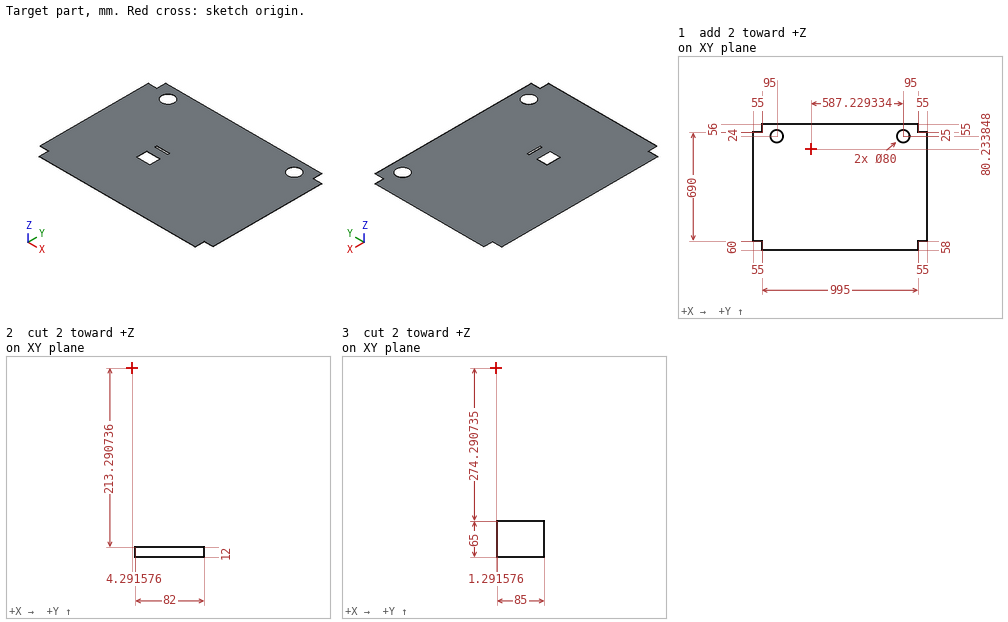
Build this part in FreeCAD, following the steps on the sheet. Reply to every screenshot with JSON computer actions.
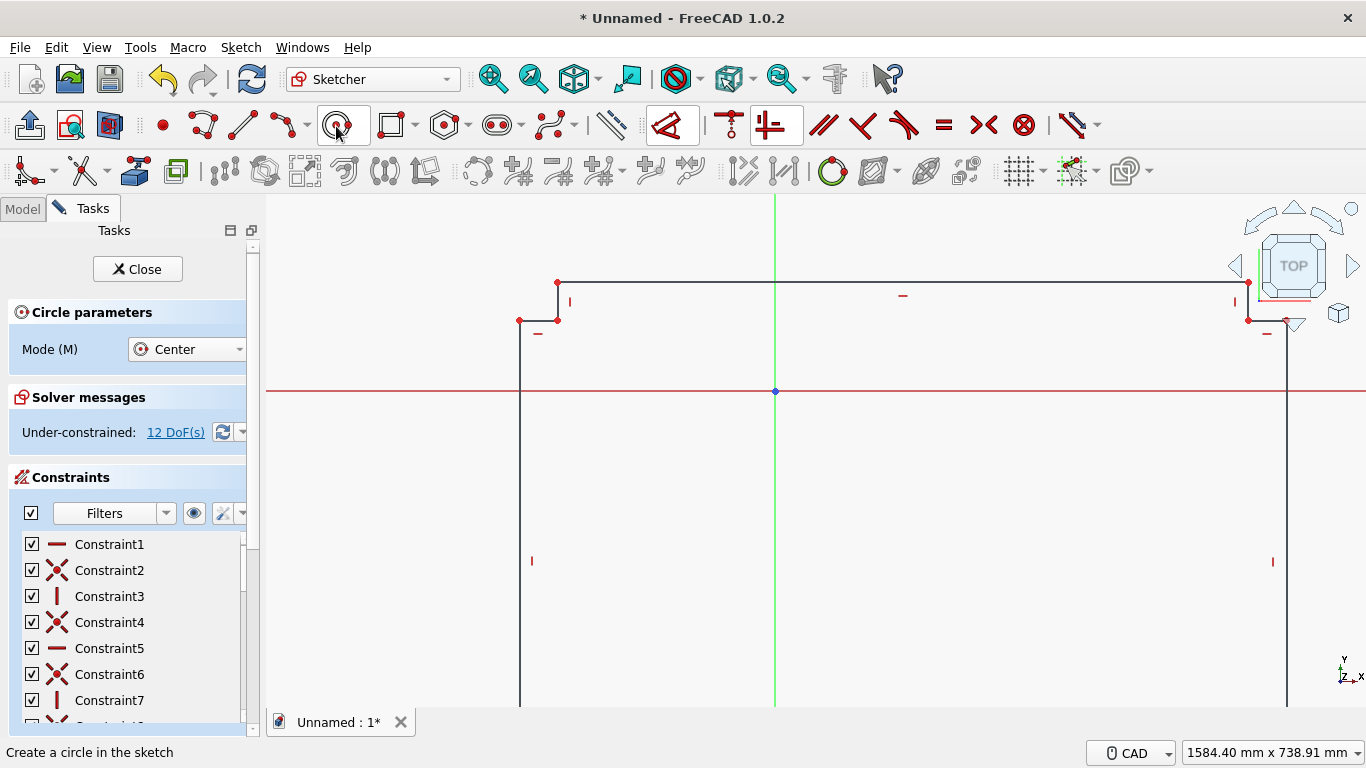
{"action": "left_click", "coordinate": [1183, 335]}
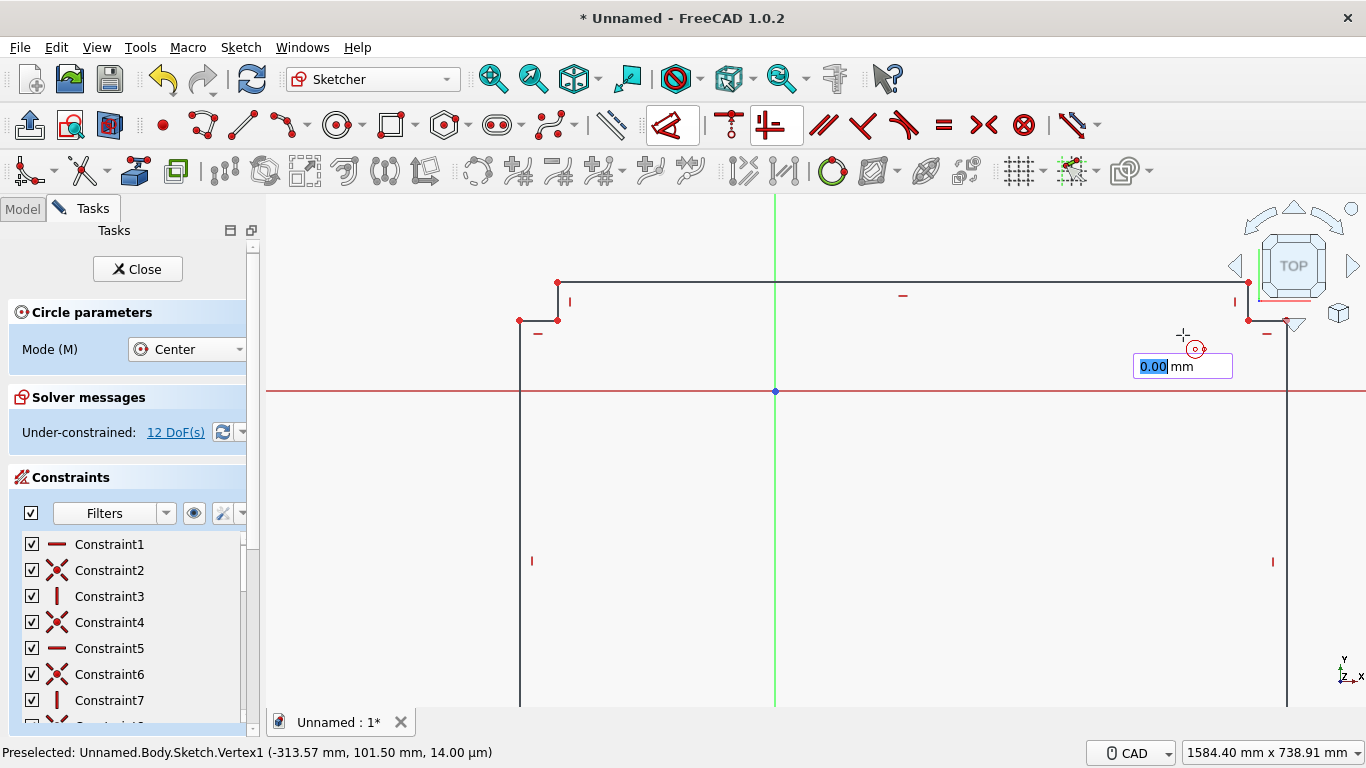
{"action": "scroll", "coordinate": [557, 318], "scroll_direction": "down", "scroll_amount": 3}
{"action": "mouse_move", "coordinate": [912, 317]}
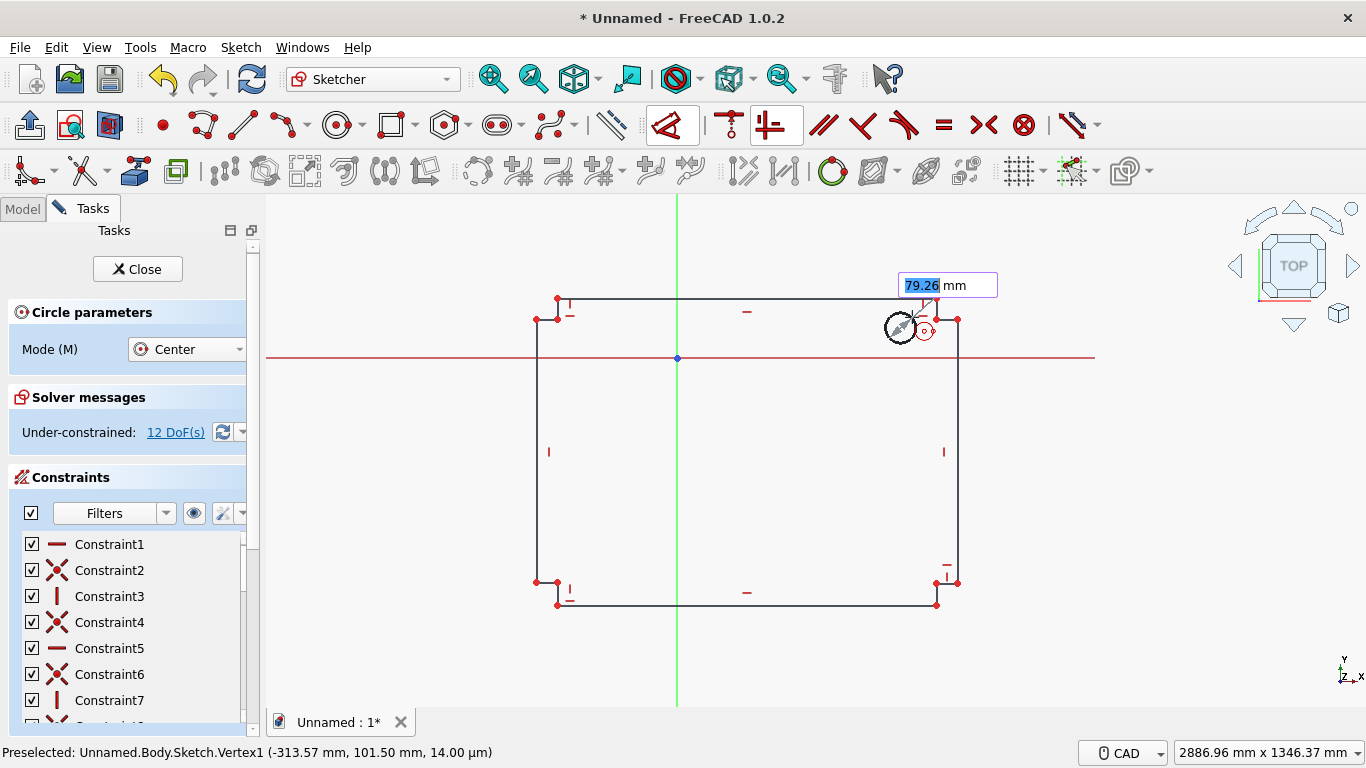
{"action": "type", "text": "80"}
{"action": "key", "text": "Return"}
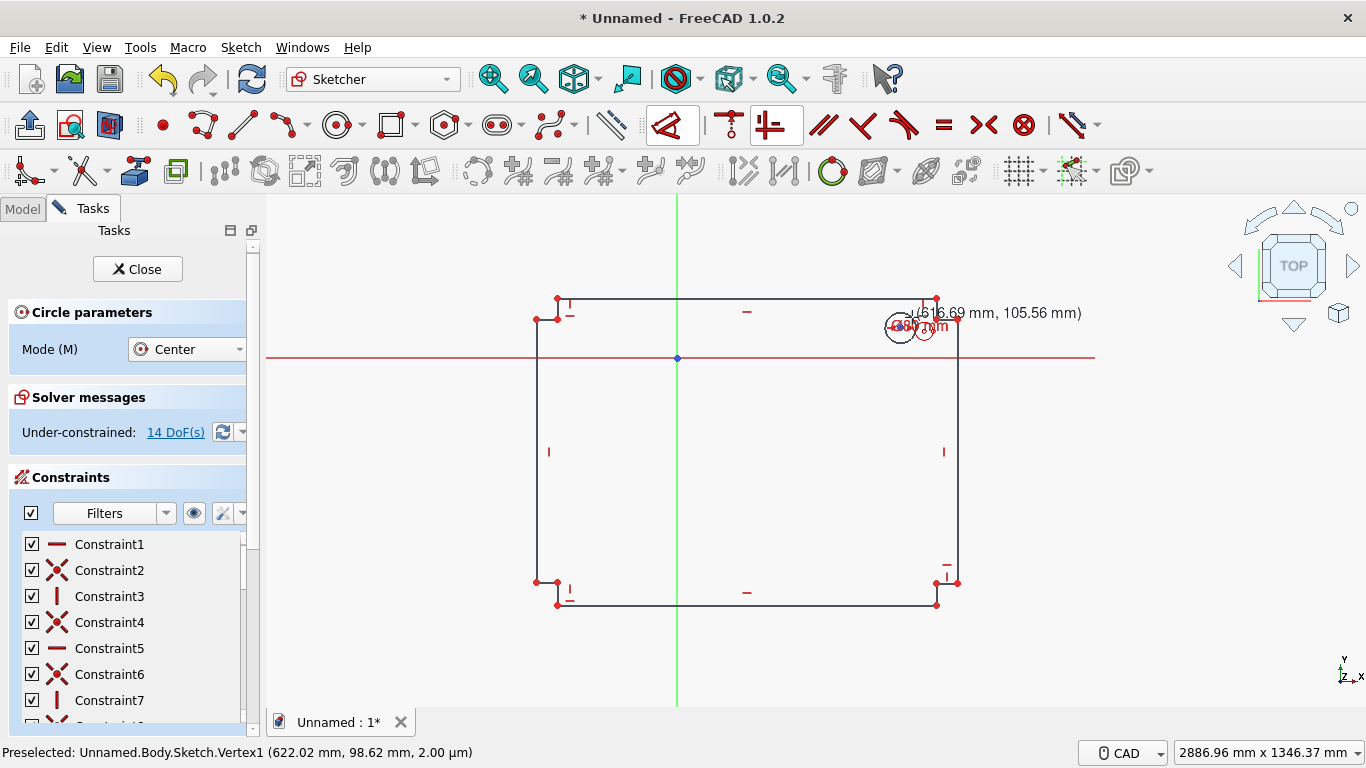
{"action": "scroll", "coordinate": [594, 328], "scroll_direction": "up", "scroll_amount": 2}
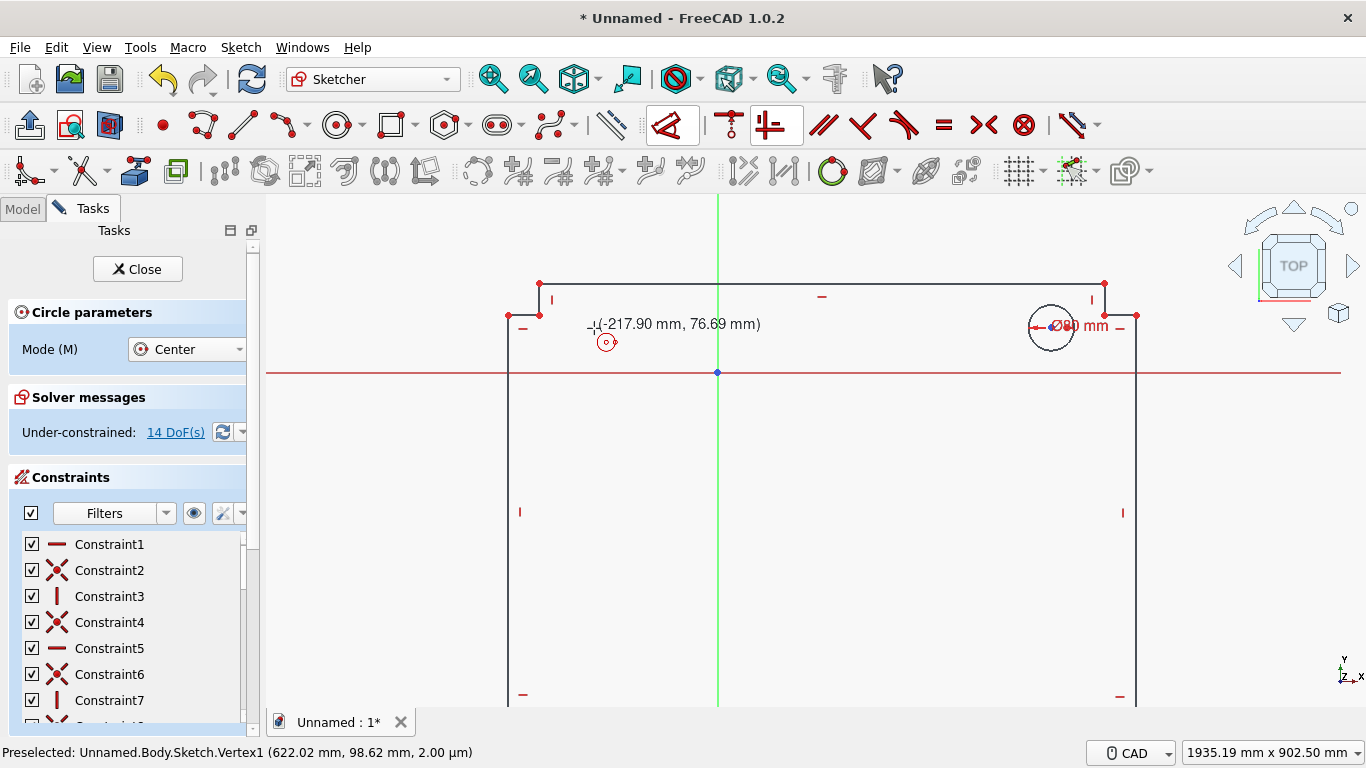
{"action": "left_click", "coordinate": [594, 327]}
{"action": "mouse_move", "coordinate": [610, 311]}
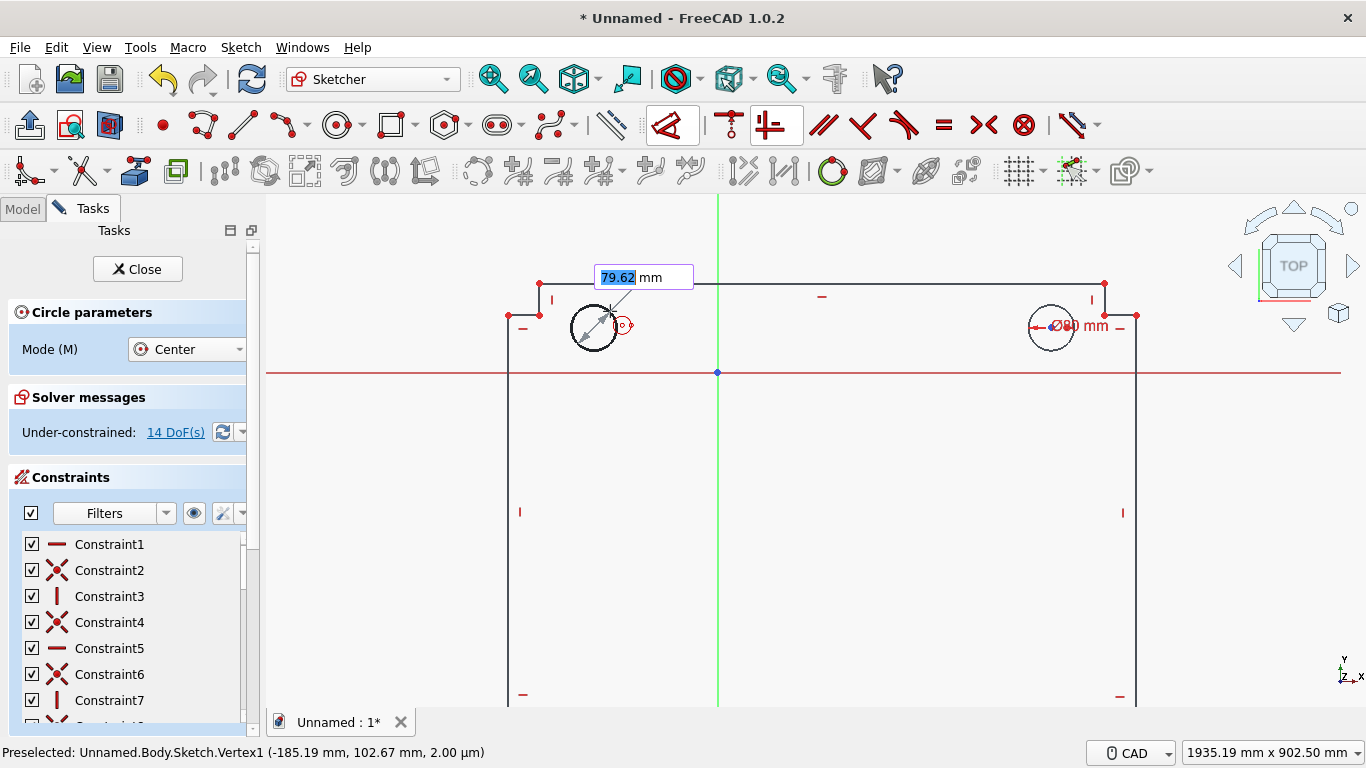
{"action": "type", "text": "80"}
{"action": "key", "text": "Return"}
{"action": "key", "text": "Escape"}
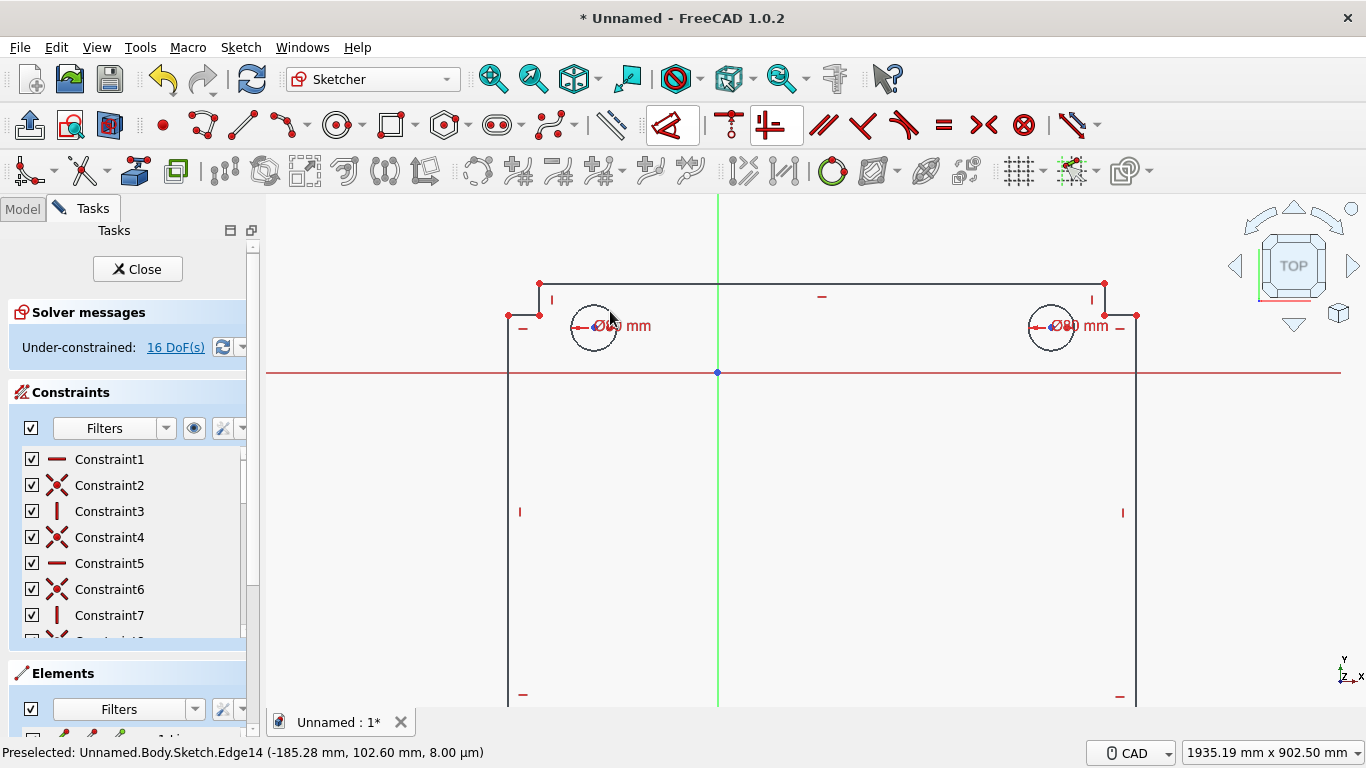
{"action": "left_click", "coordinate": [666, 126]}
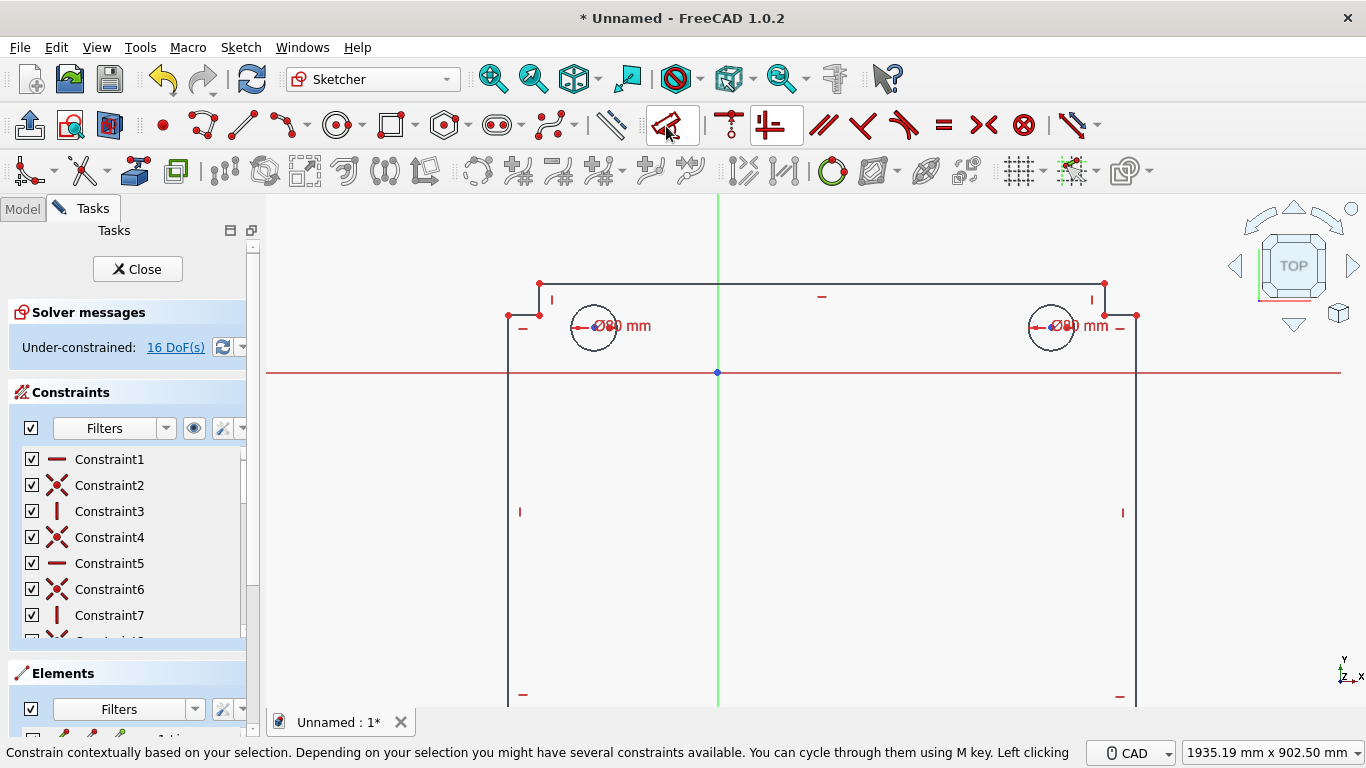
{"action": "scroll", "coordinate": [530, 315], "scroll_direction": "up", "scroll_amount": 2}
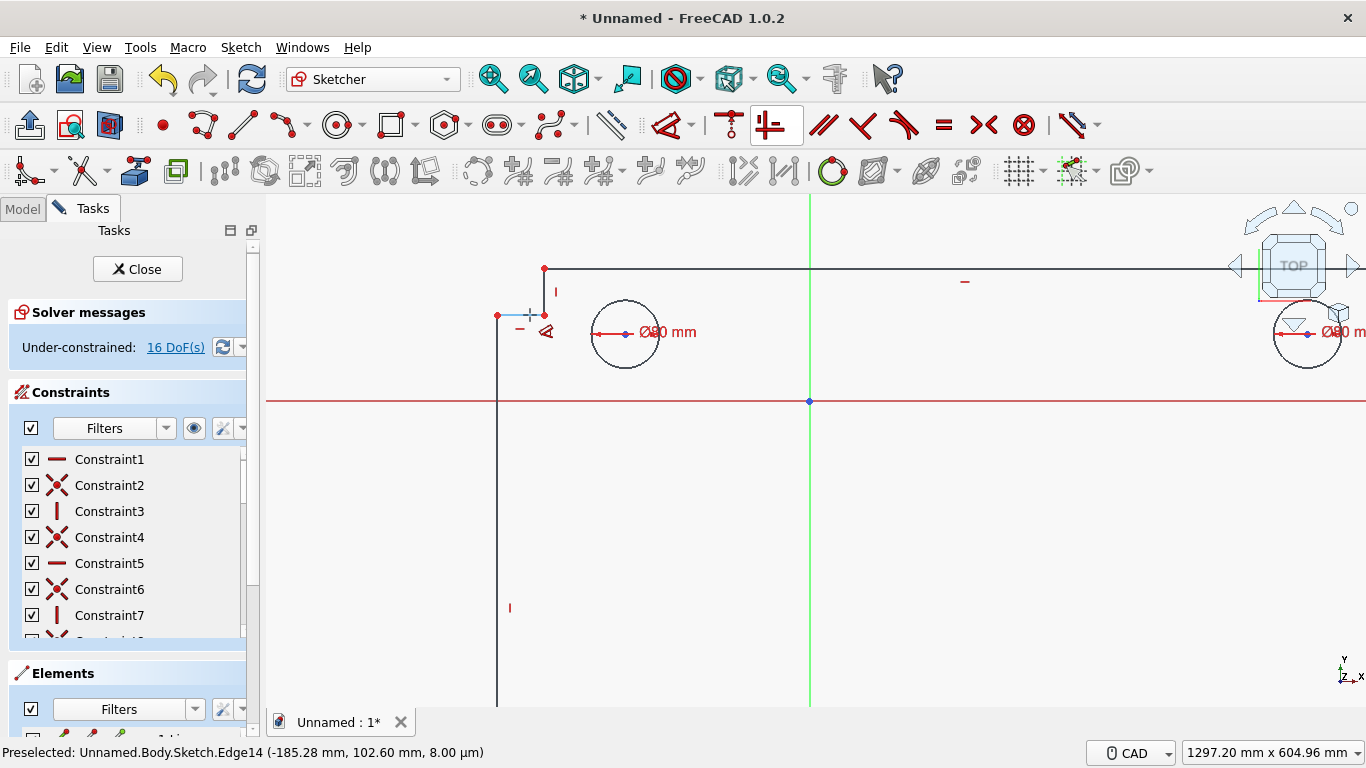
{"action": "left_click", "coordinate": [530, 315]}
{"action": "left_click", "coordinate": [521, 281]}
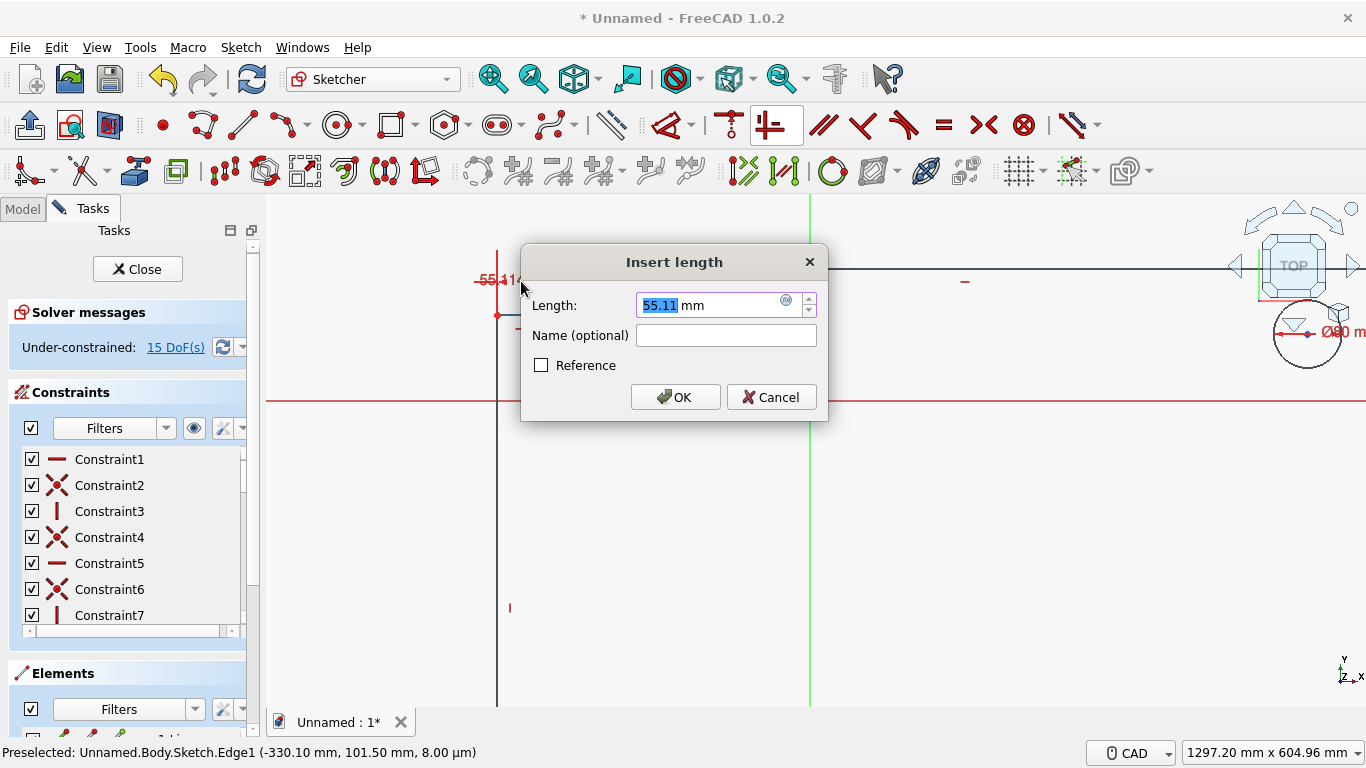
{"action": "type", "text": "55"}
{"action": "key", "text": "Return"}